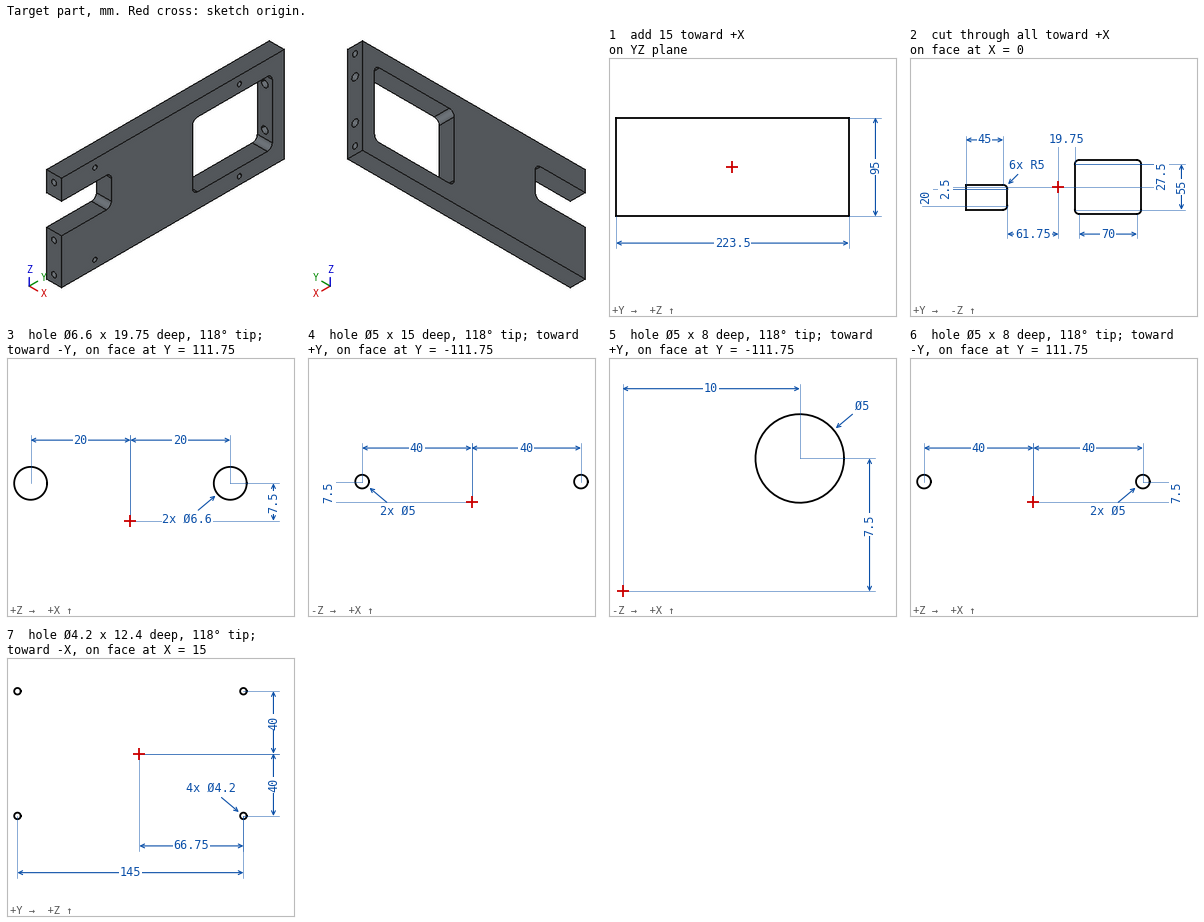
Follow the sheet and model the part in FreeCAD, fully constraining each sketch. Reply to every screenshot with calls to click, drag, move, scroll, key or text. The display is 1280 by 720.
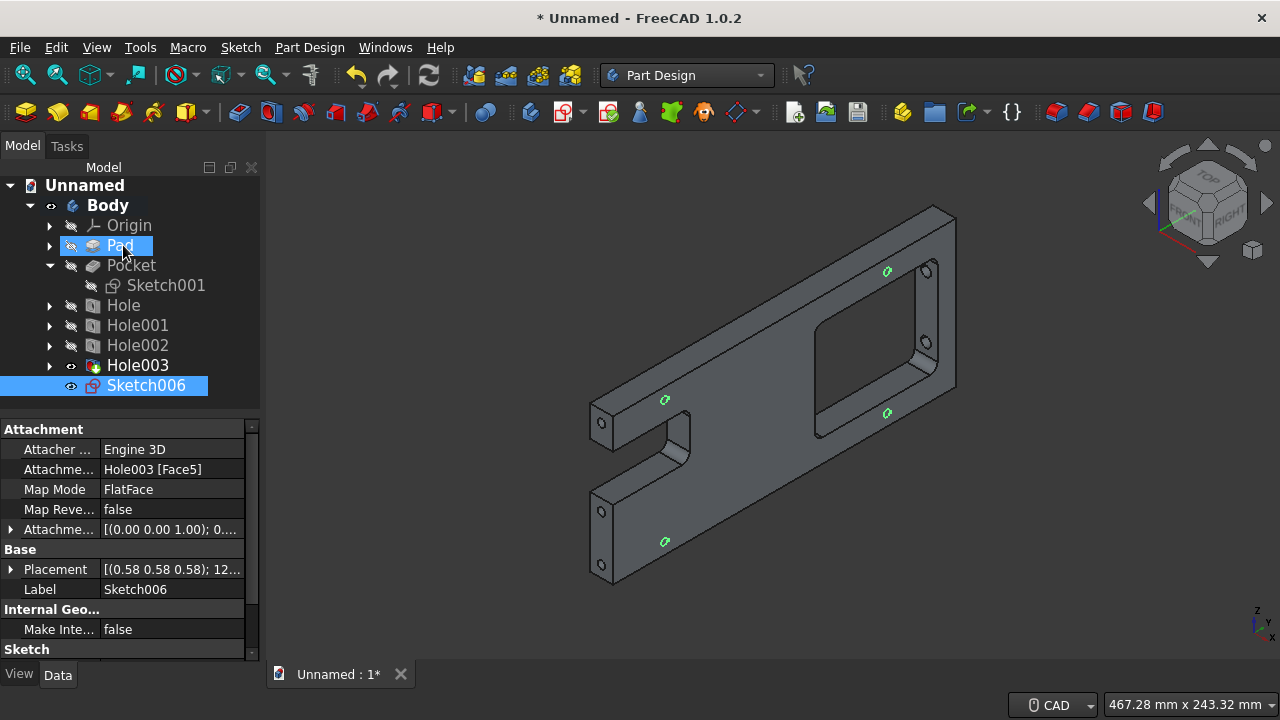
click(272, 112)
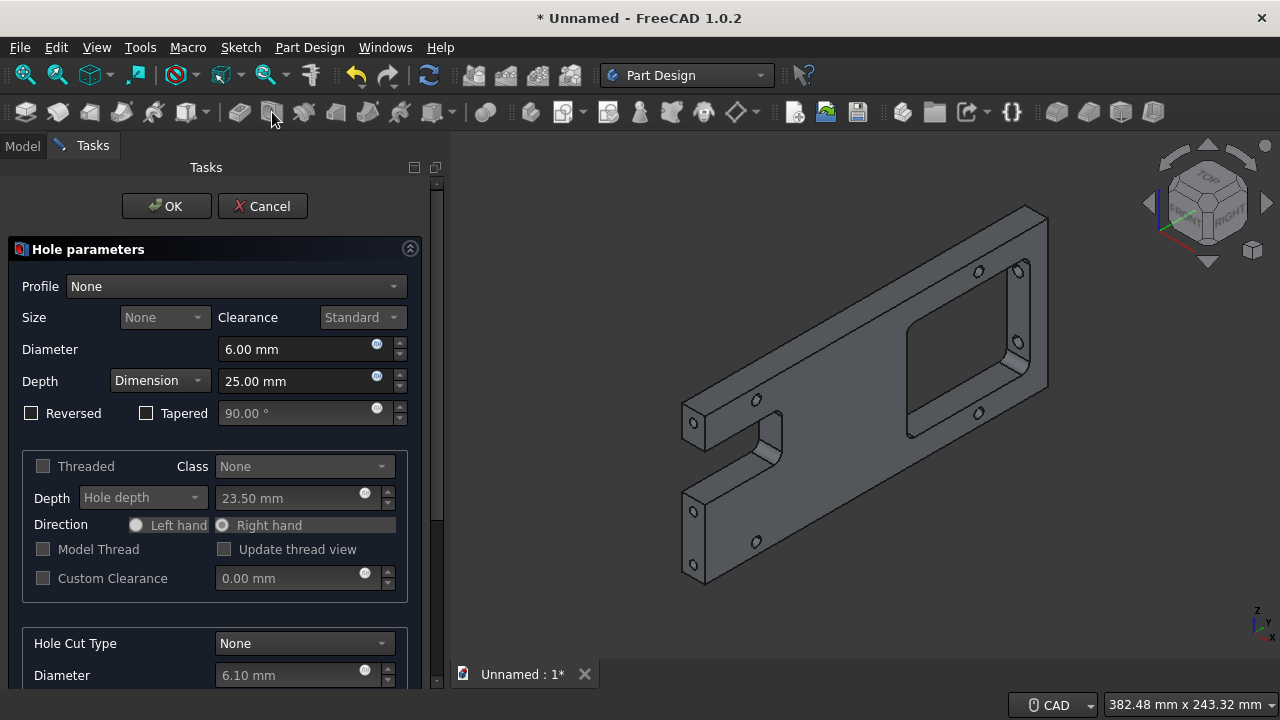
triple_click(305, 349)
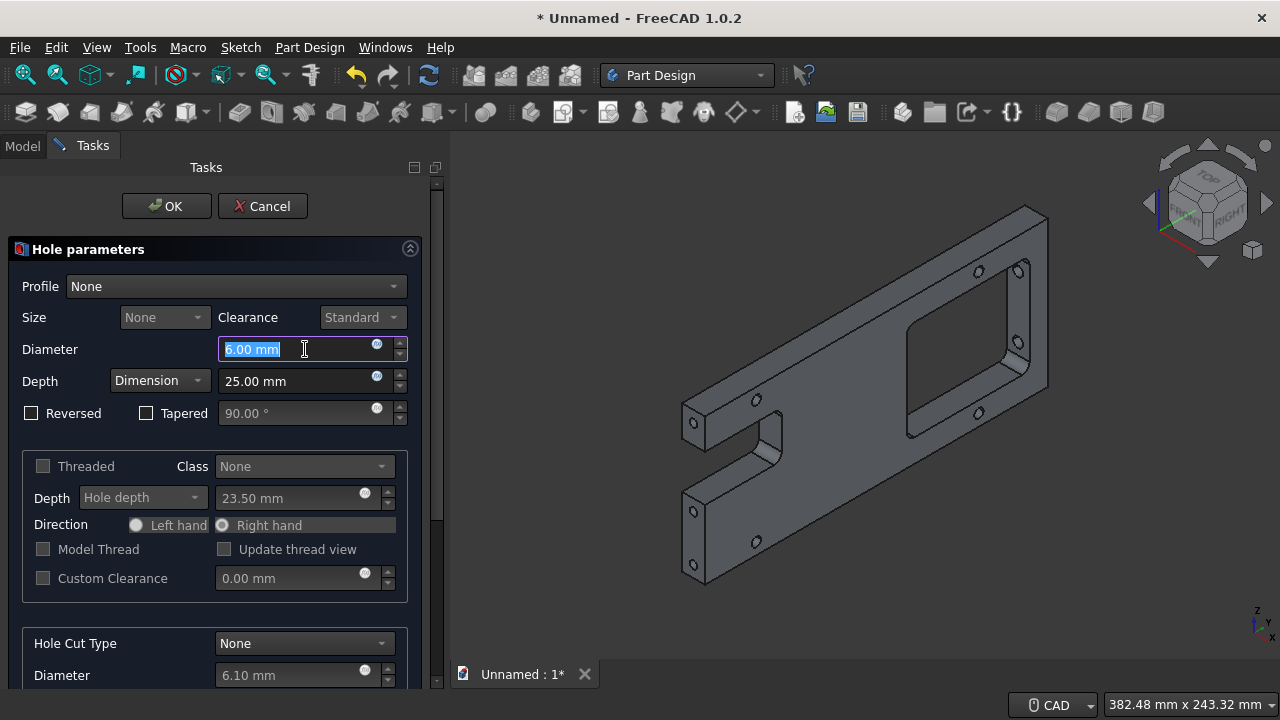
text(4.2)
key(Tab)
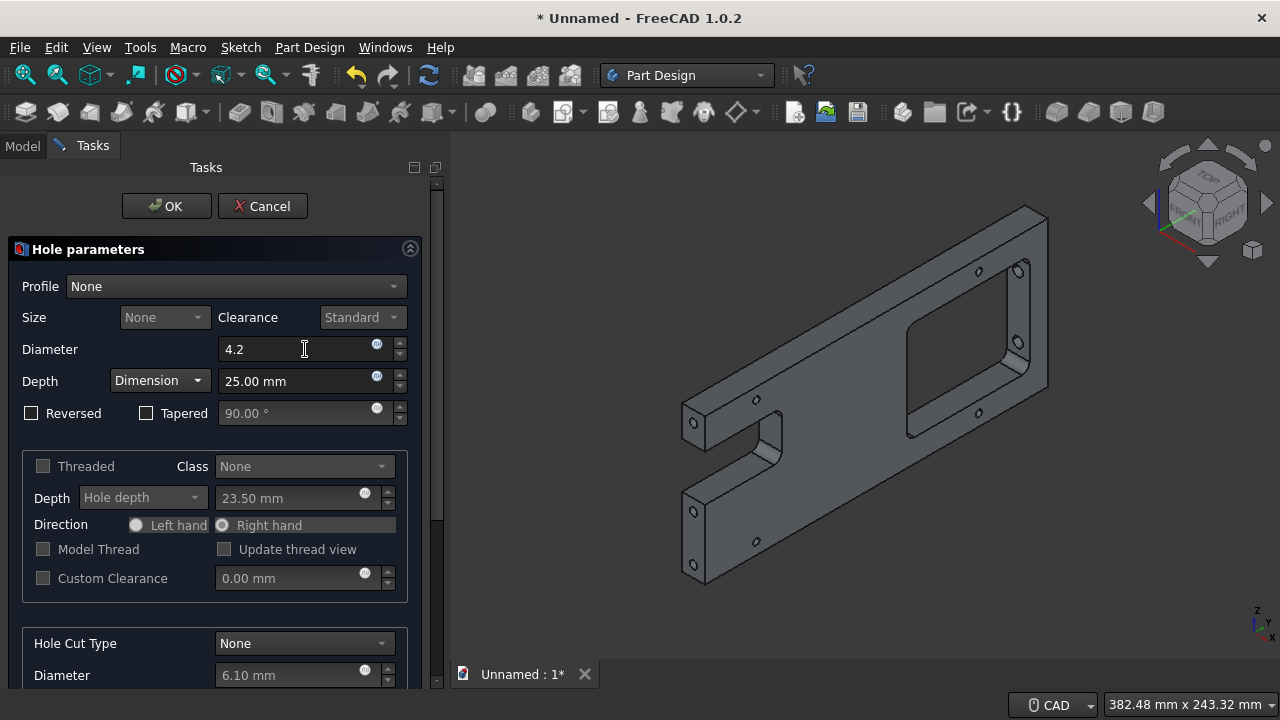
triple_click(305, 381)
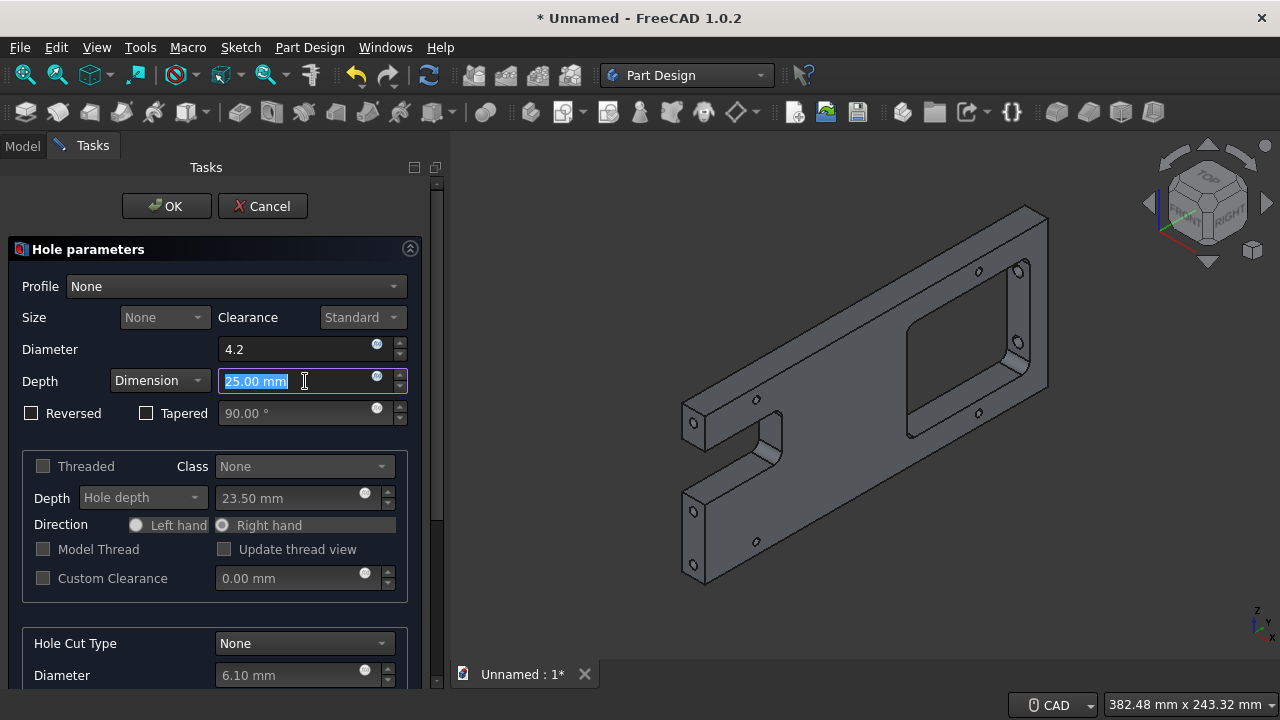
text(12.4)
key(Tab)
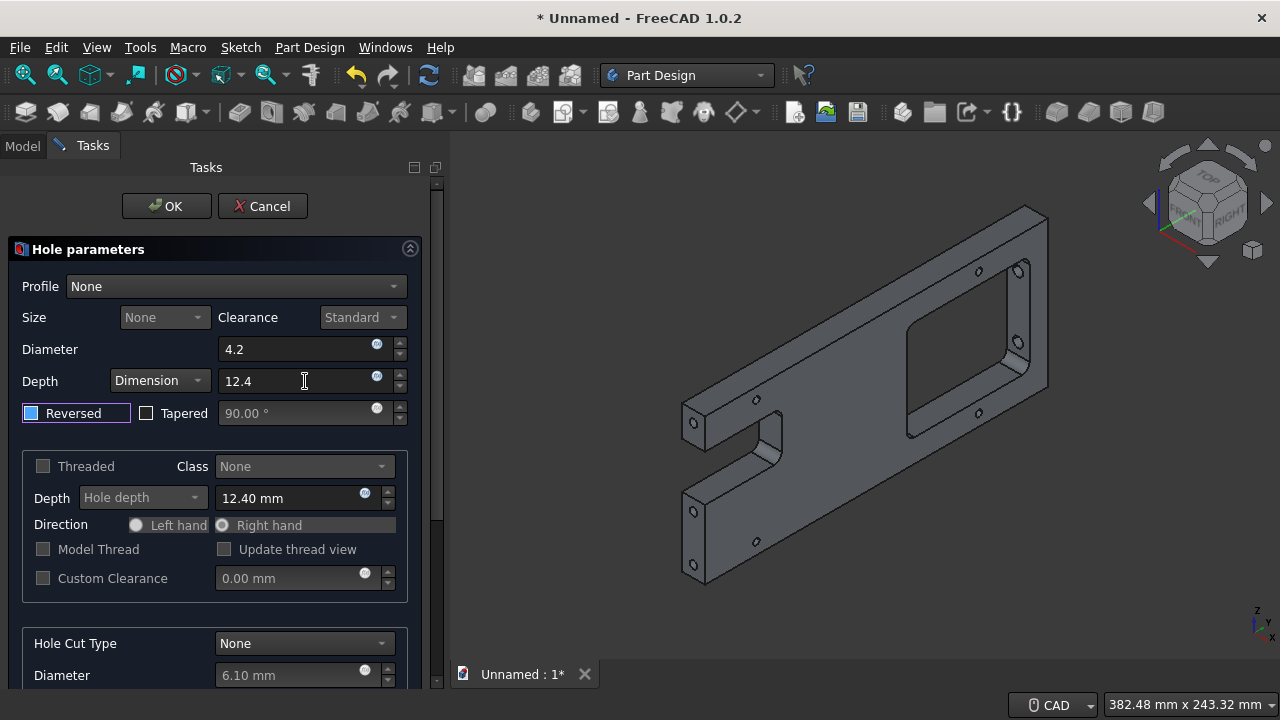
click(167, 206)